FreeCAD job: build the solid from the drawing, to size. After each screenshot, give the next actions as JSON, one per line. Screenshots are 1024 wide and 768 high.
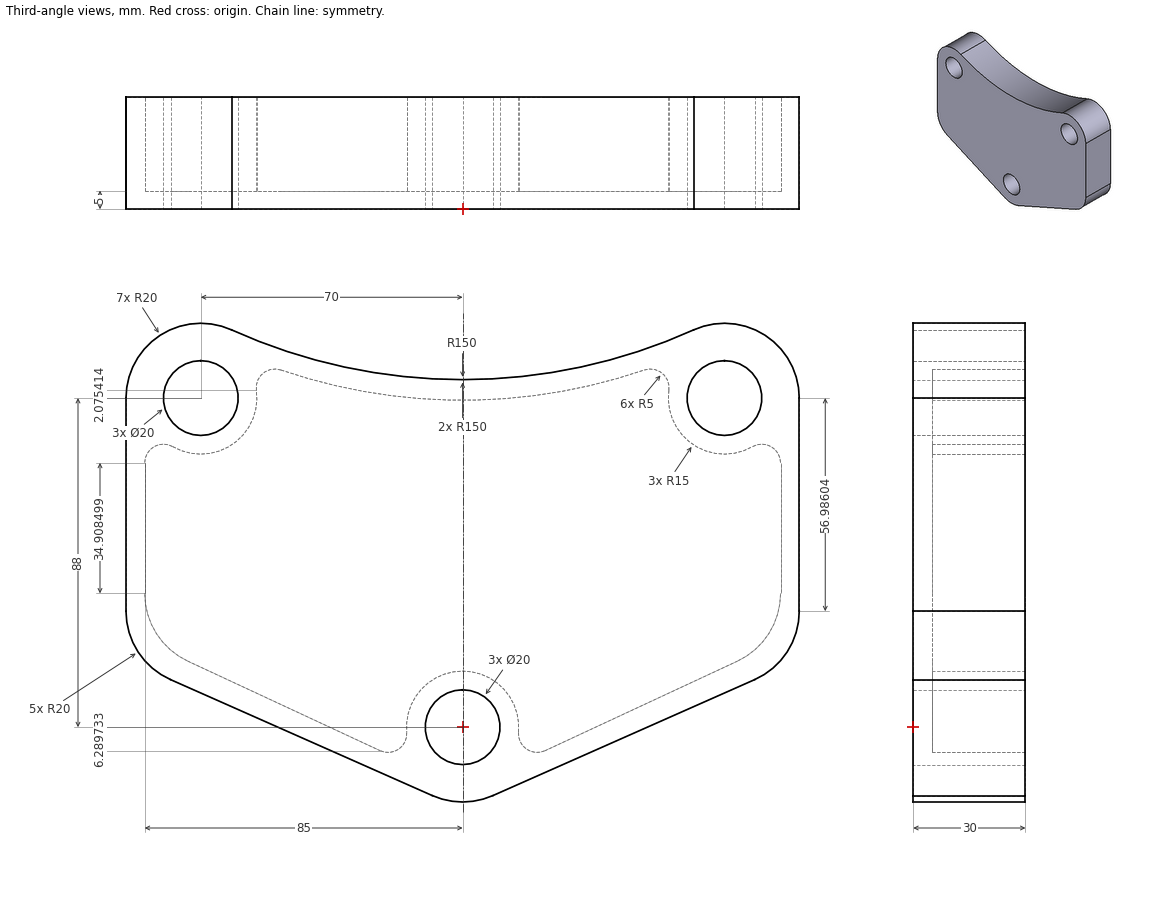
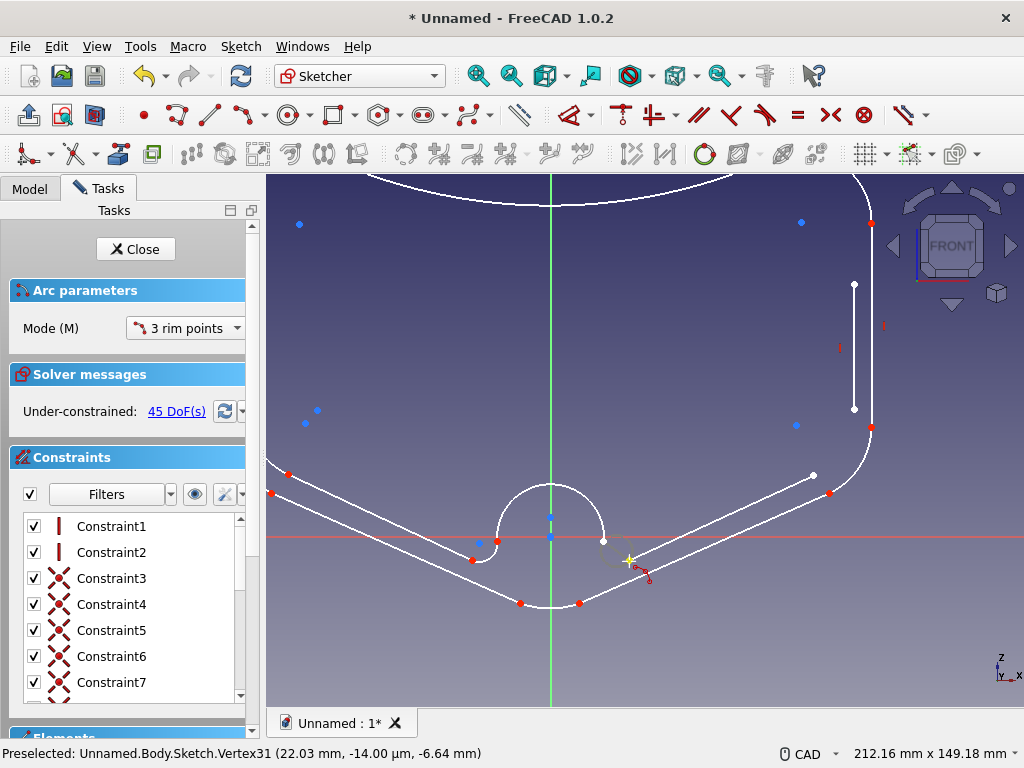
{"action": "scroll", "coordinate": [612, 558], "scroll_direction": "up", "scroll_amount": 3}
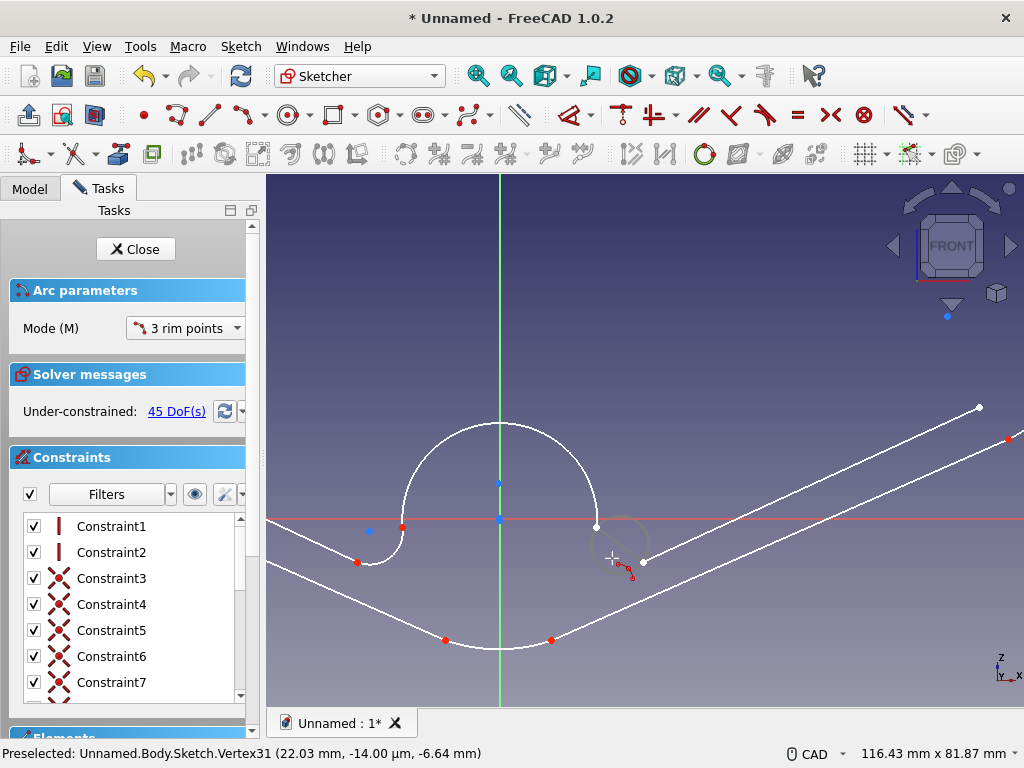
{"action": "left_click", "coordinate": [611, 557]}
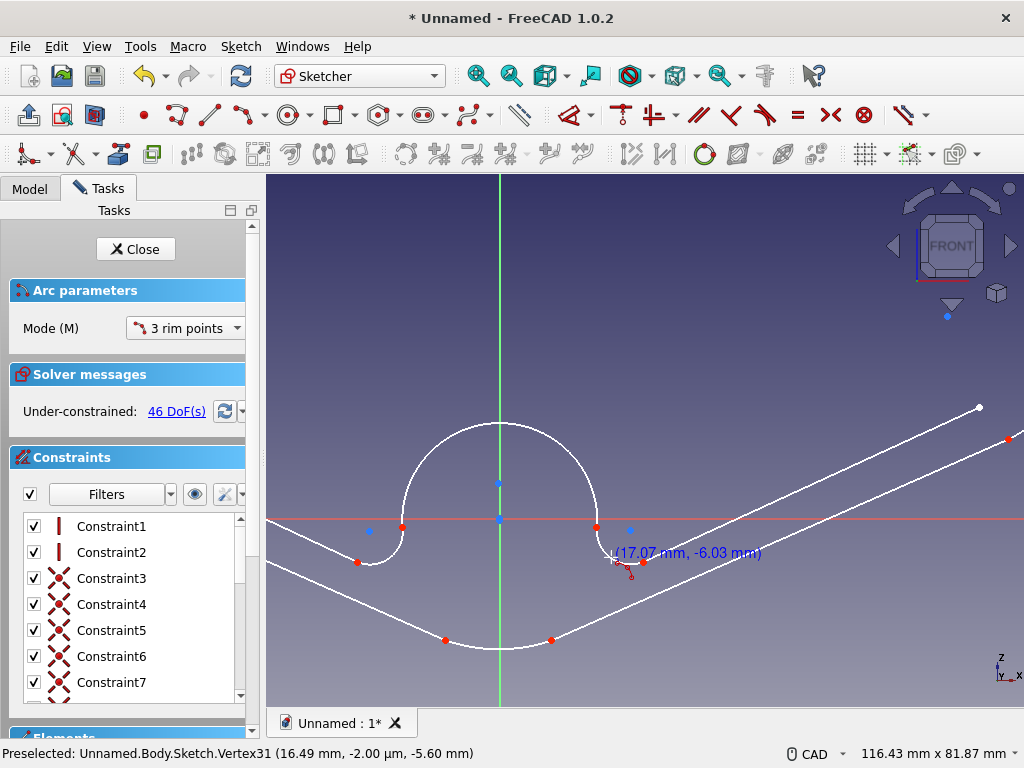
{"action": "scroll", "coordinate": [621, 558], "scroll_direction": "down", "scroll_amount": 5}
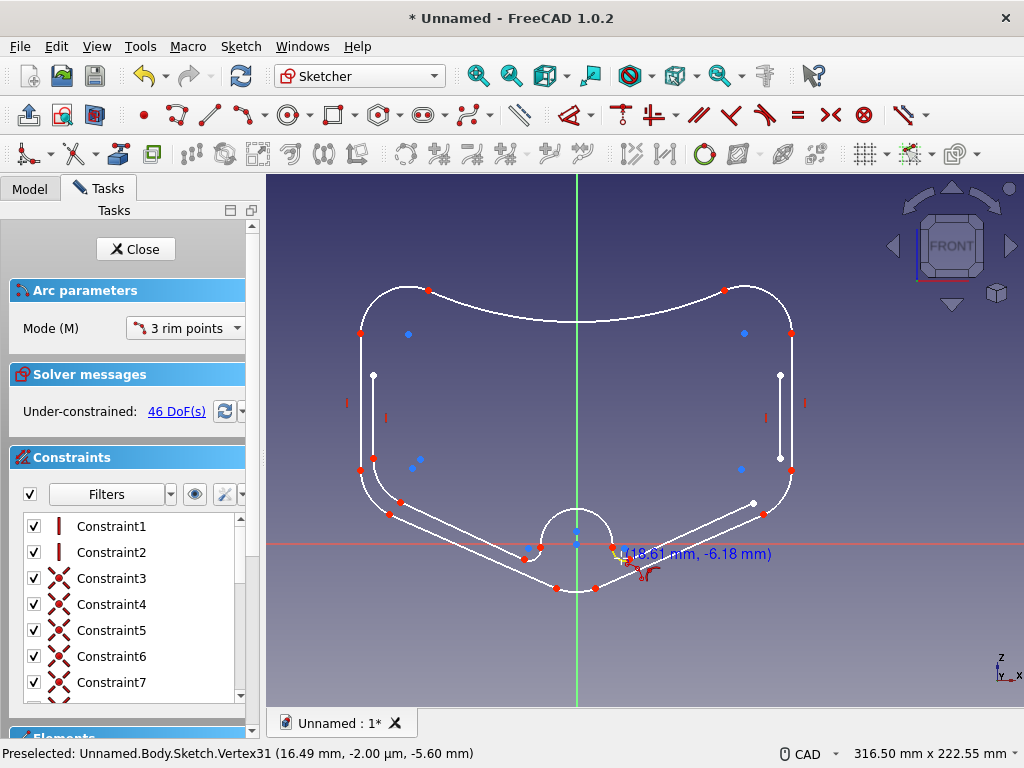
{"action": "left_click", "coordinate": [753, 503]}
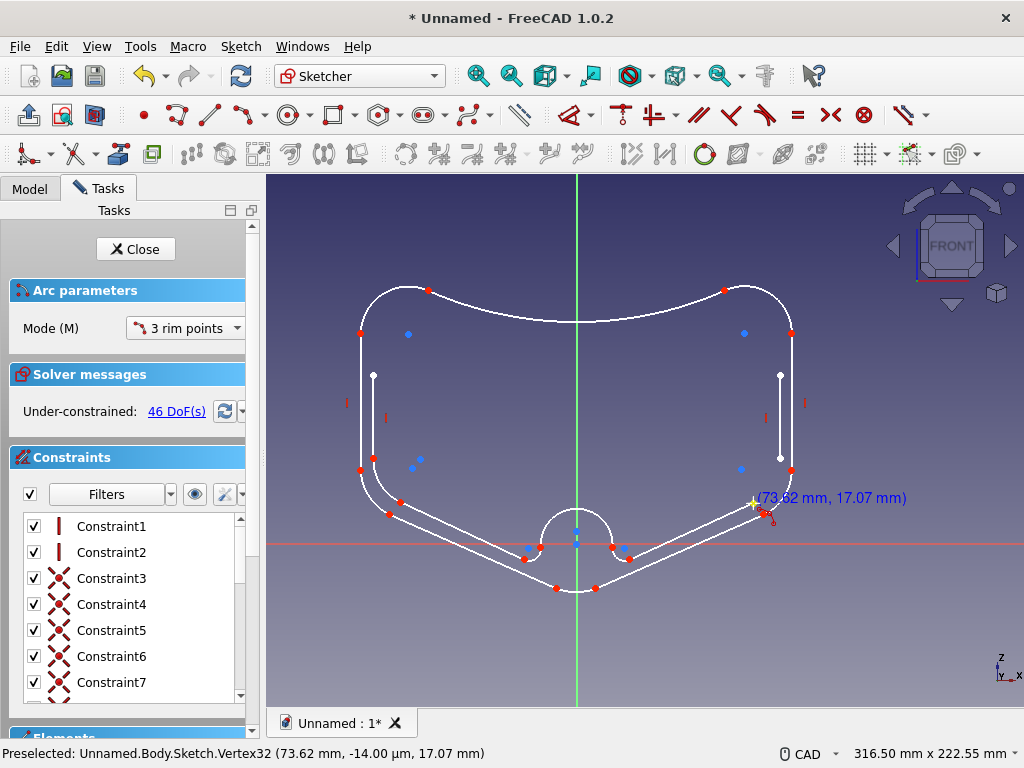
{"action": "scroll", "coordinate": [780, 458], "scroll_direction": "up", "scroll_amount": 2}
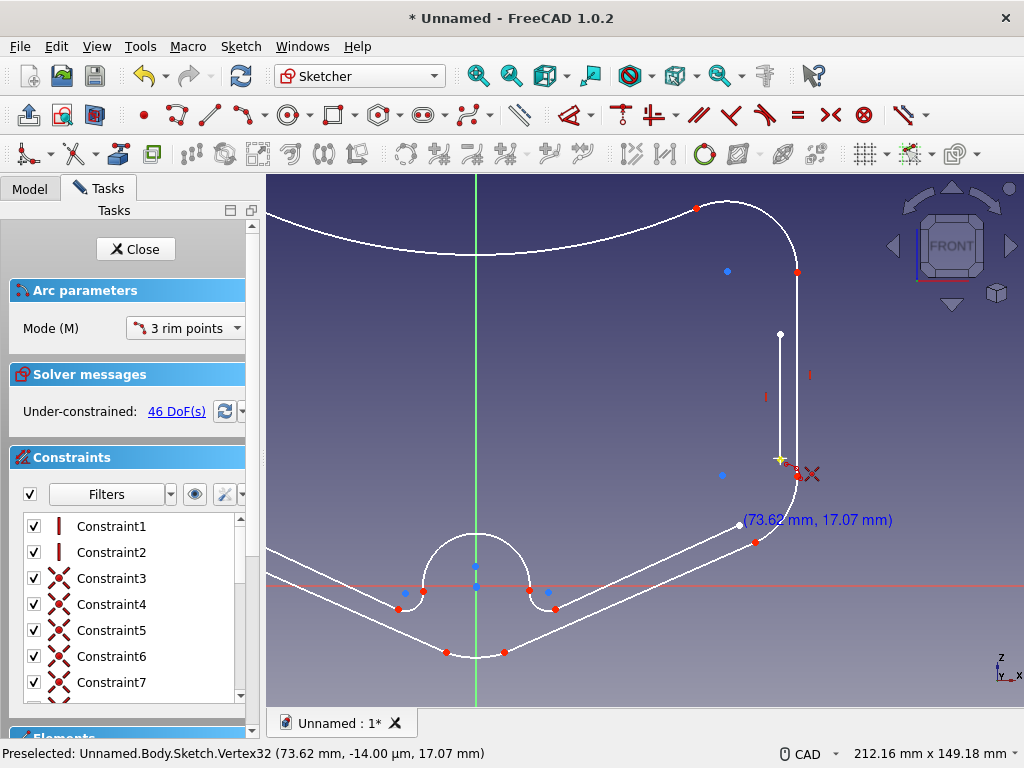
{"action": "left_click", "coordinate": [780, 459]}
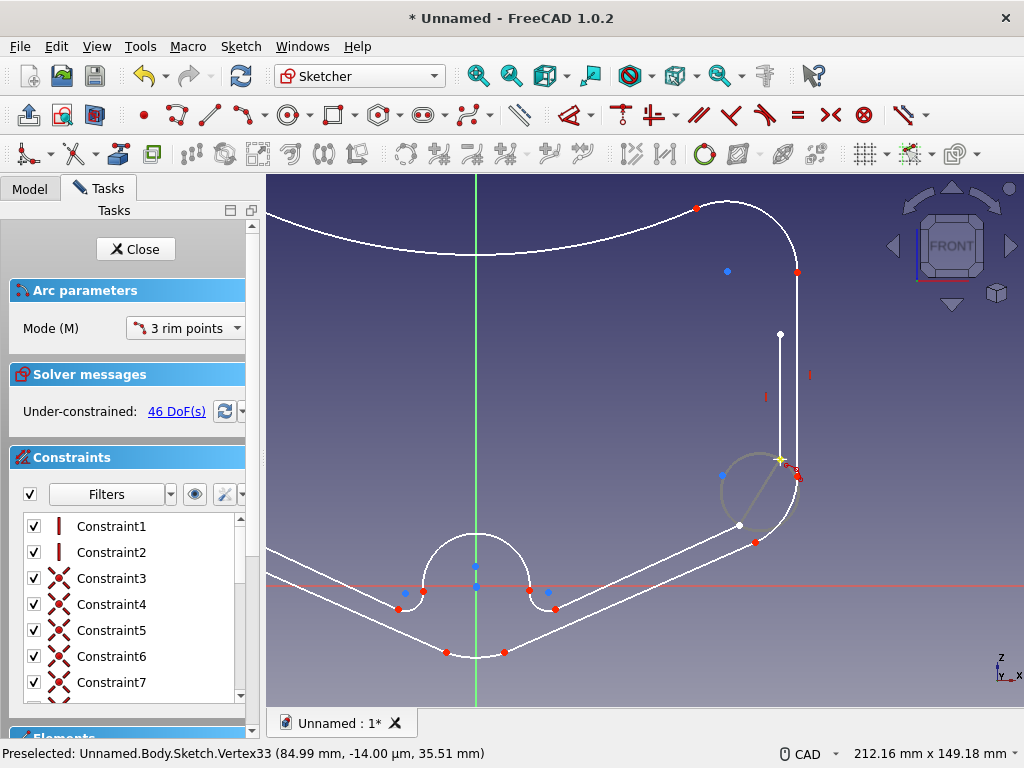
{"action": "scroll", "coordinate": [769, 497], "scroll_direction": "up", "scroll_amount": 2}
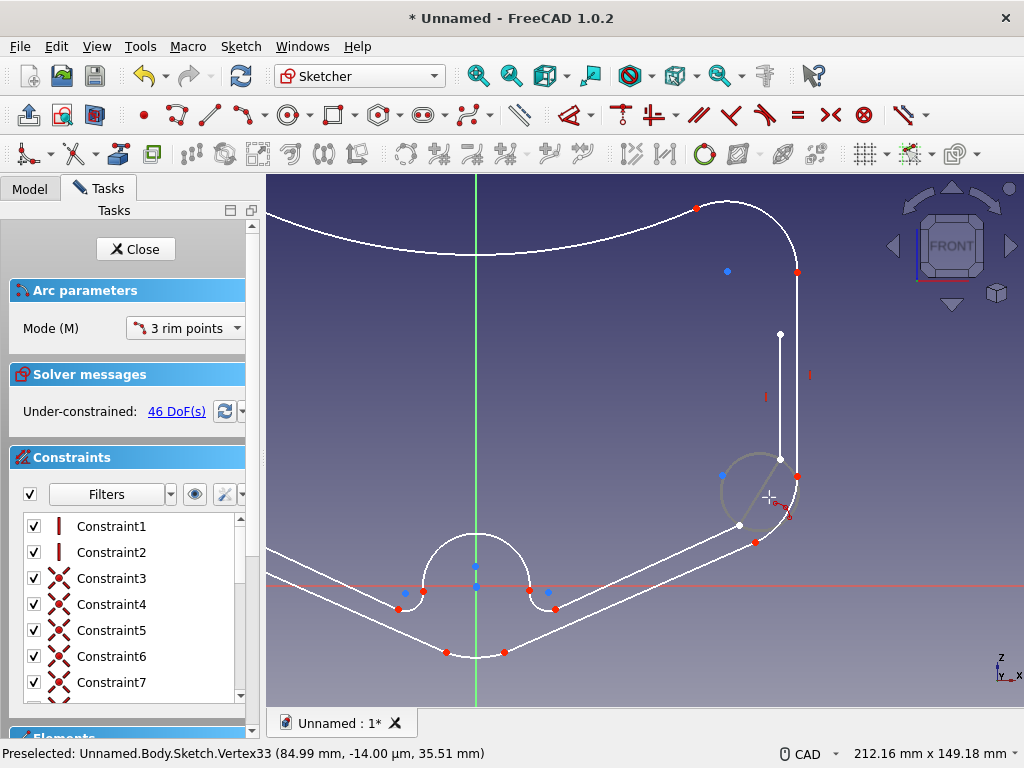
{"action": "left_click", "coordinate": [769, 496]}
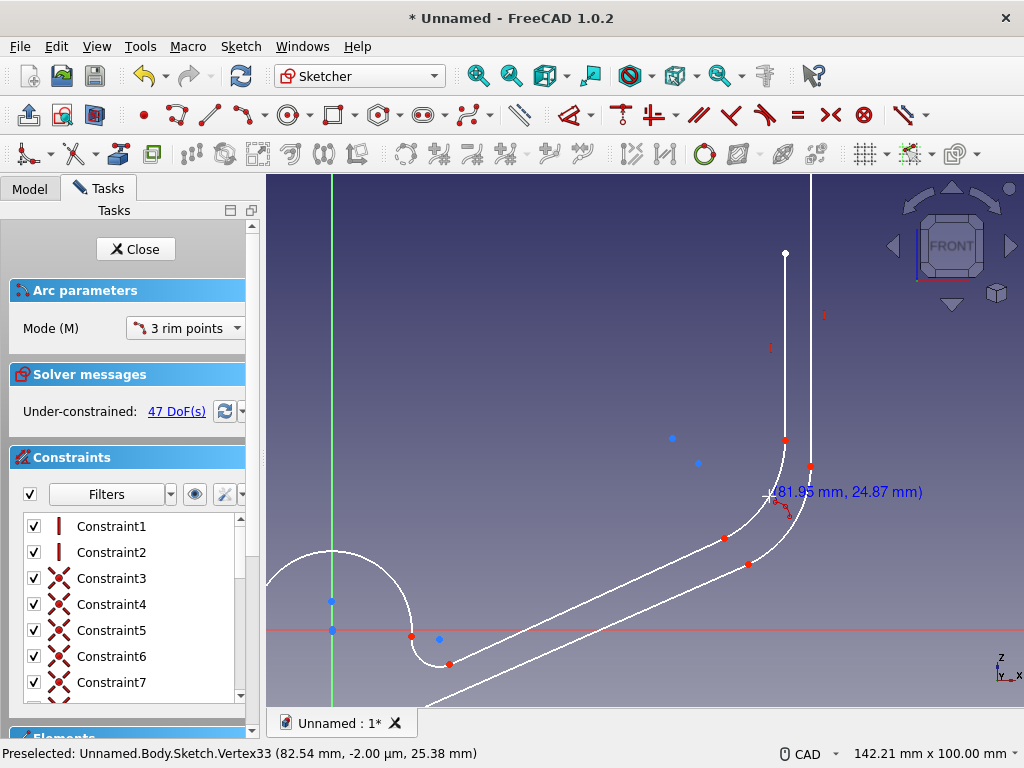
{"action": "left_click", "coordinate": [785, 254]}
{"action": "left_click", "coordinate": [745, 230]}
{"action": "left_click", "coordinate": [772, 230]}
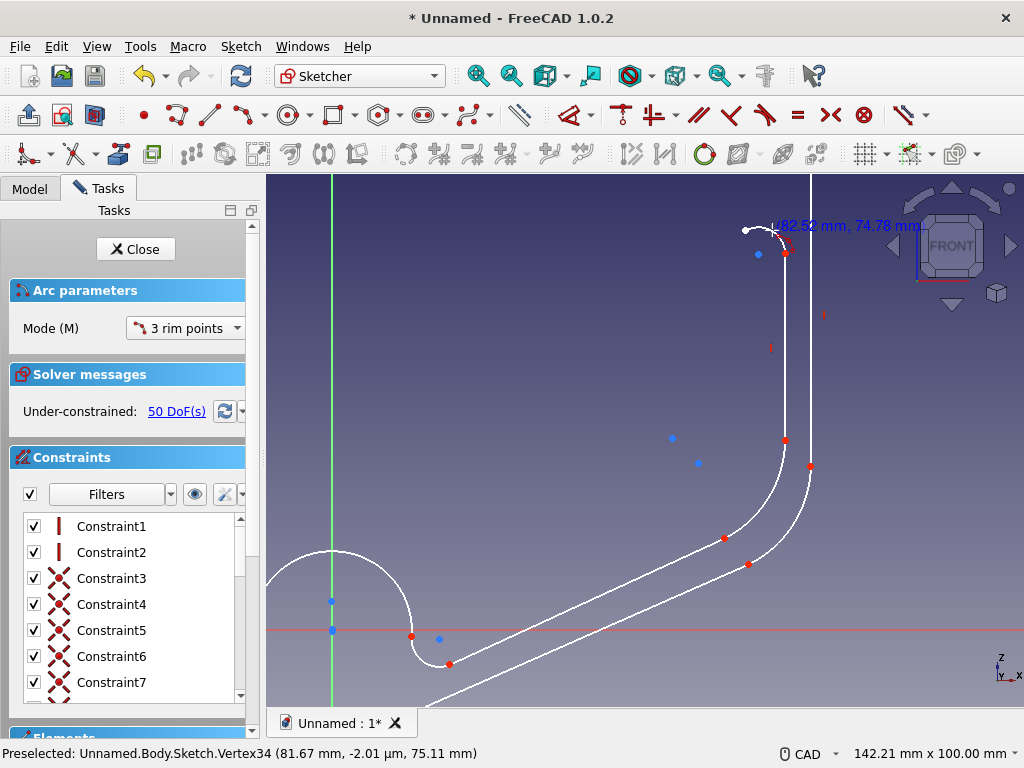
{"action": "left_click", "coordinate": [745, 231]}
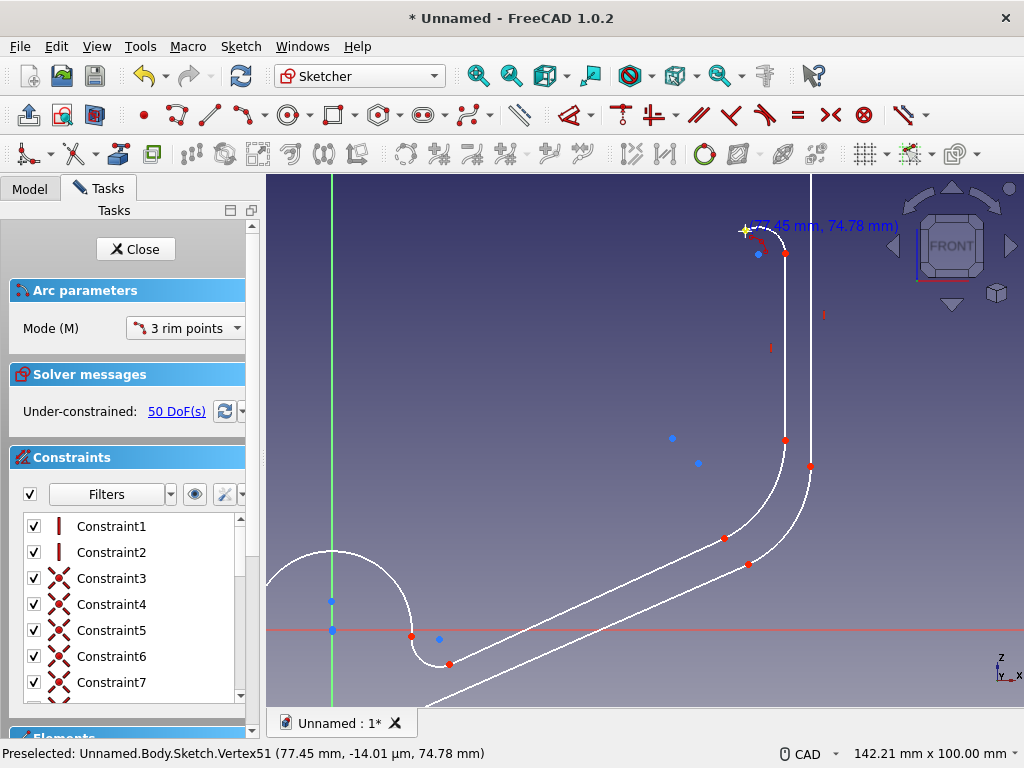
{"action": "scroll", "coordinate": [776, 474], "scroll_direction": "down", "scroll_amount": 4}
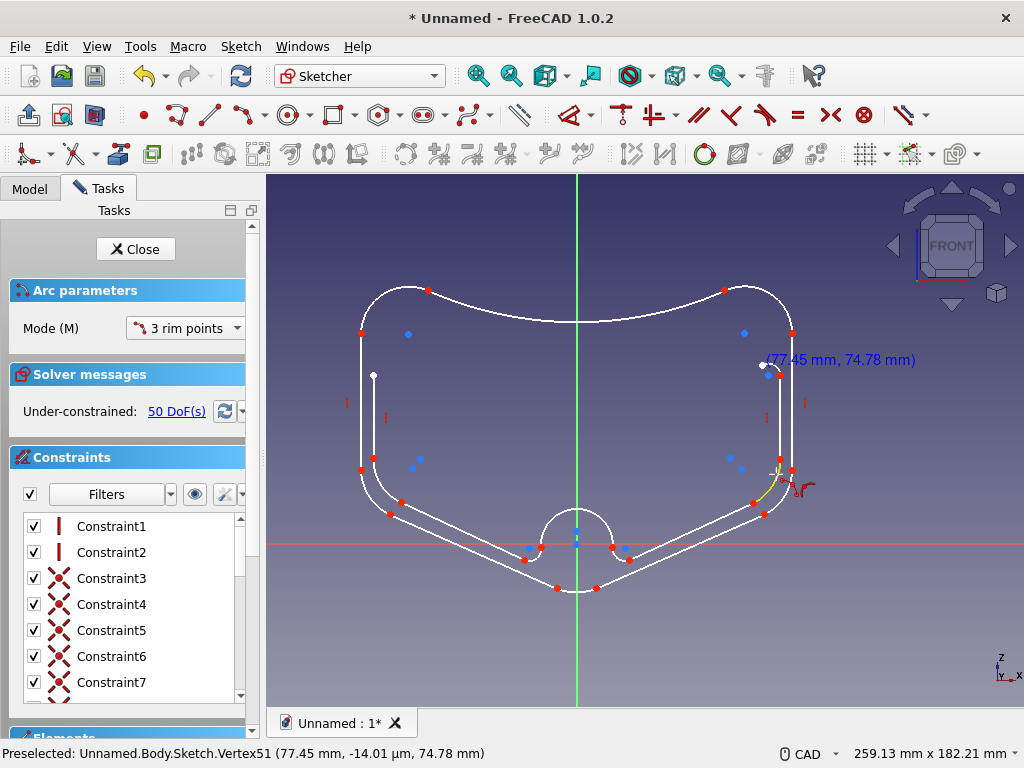
{"action": "left_click", "coordinate": [709, 328]}
{"action": "left_click", "coordinate": [725, 363]}